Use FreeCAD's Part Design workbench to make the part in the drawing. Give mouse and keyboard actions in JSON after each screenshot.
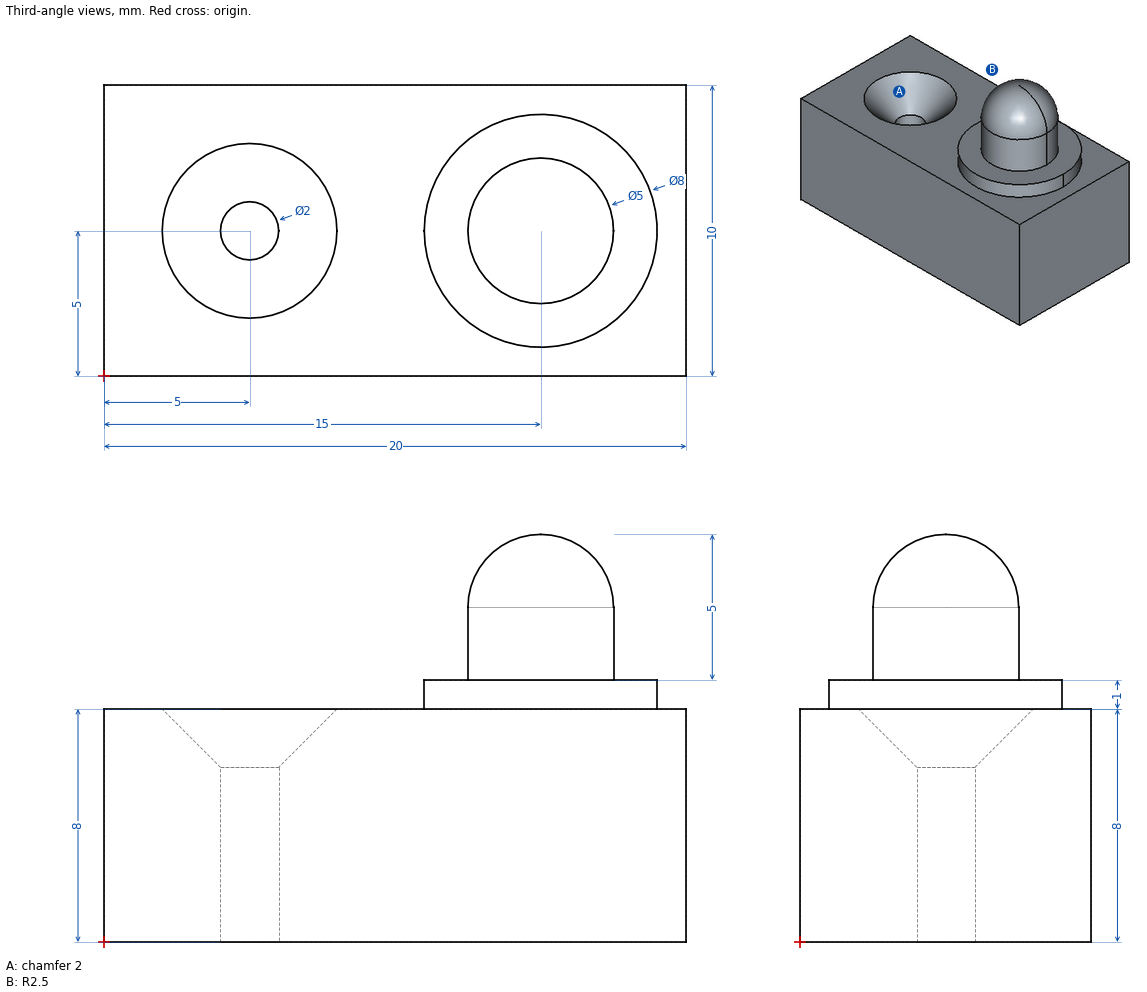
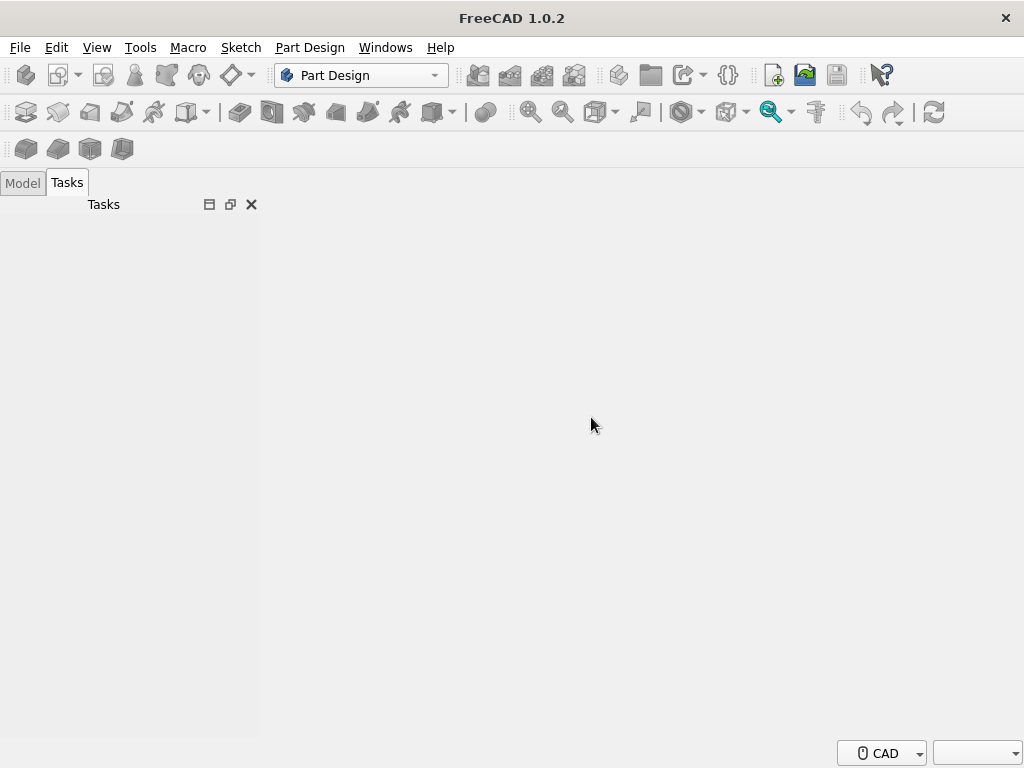
{"action": "left_click", "coordinate": [774, 76]}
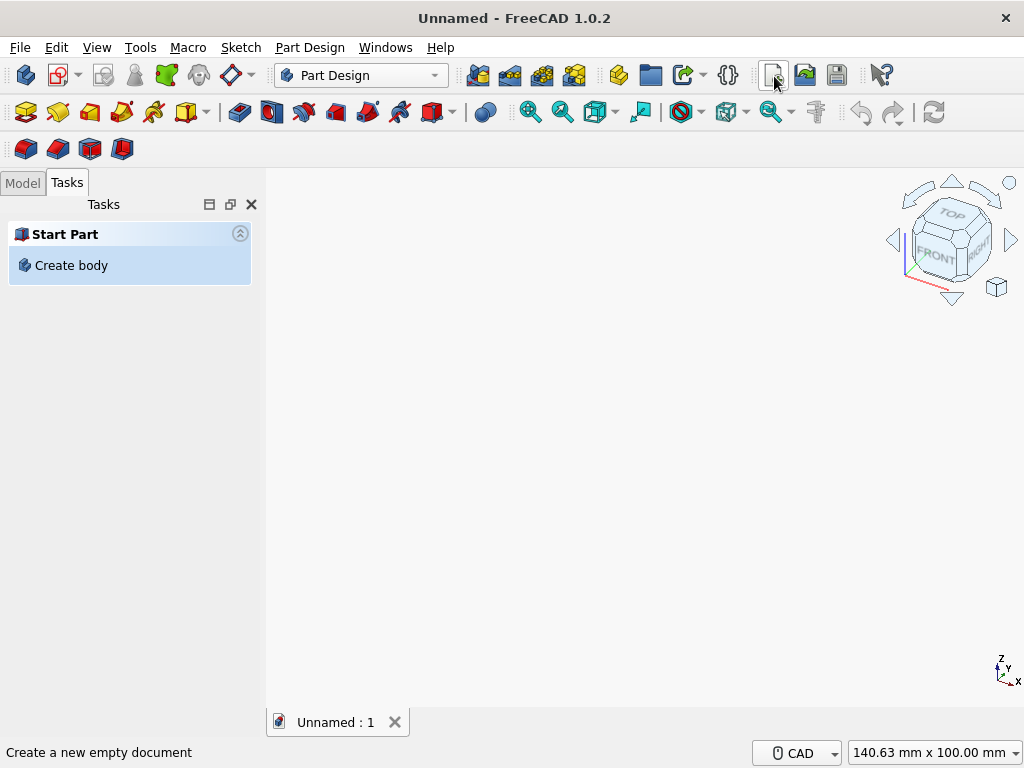
{"action": "left_click", "coordinate": [58, 76]}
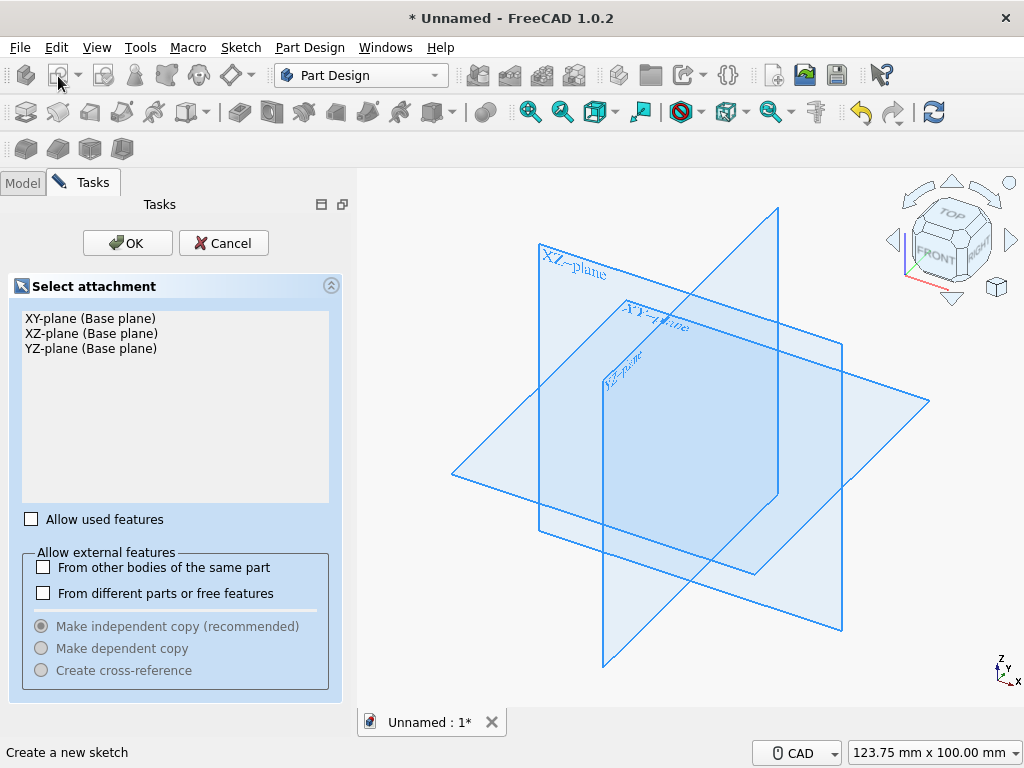
{"action": "left_click", "coordinate": [82, 318]}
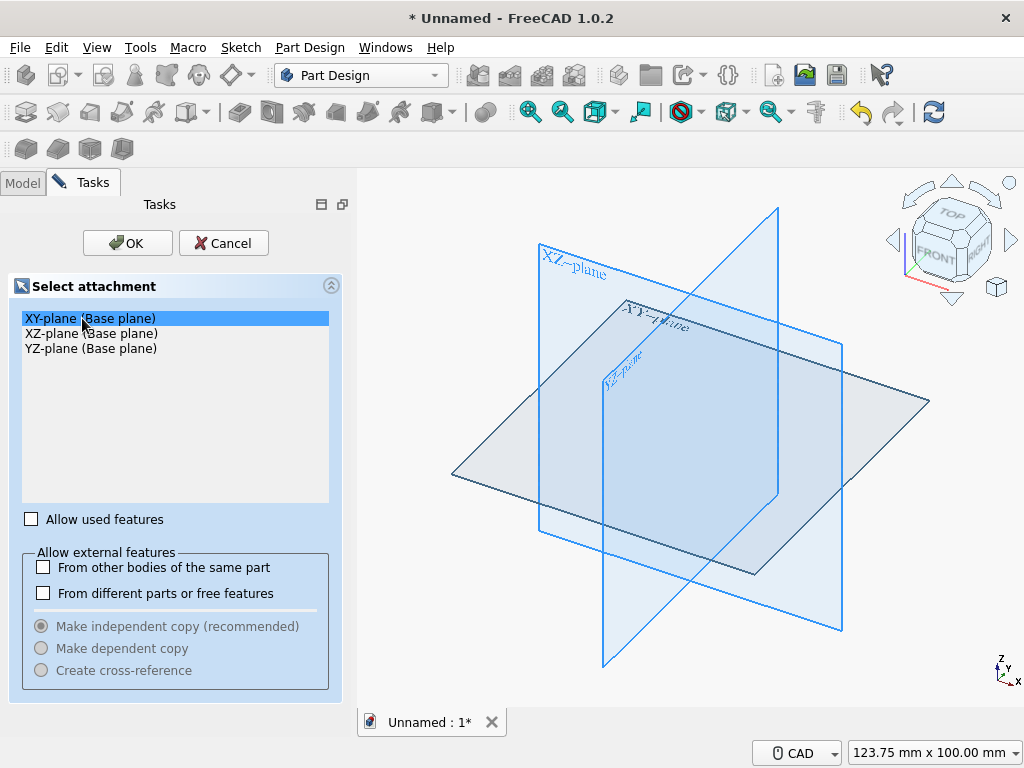
{"action": "left_click", "coordinate": [128, 243]}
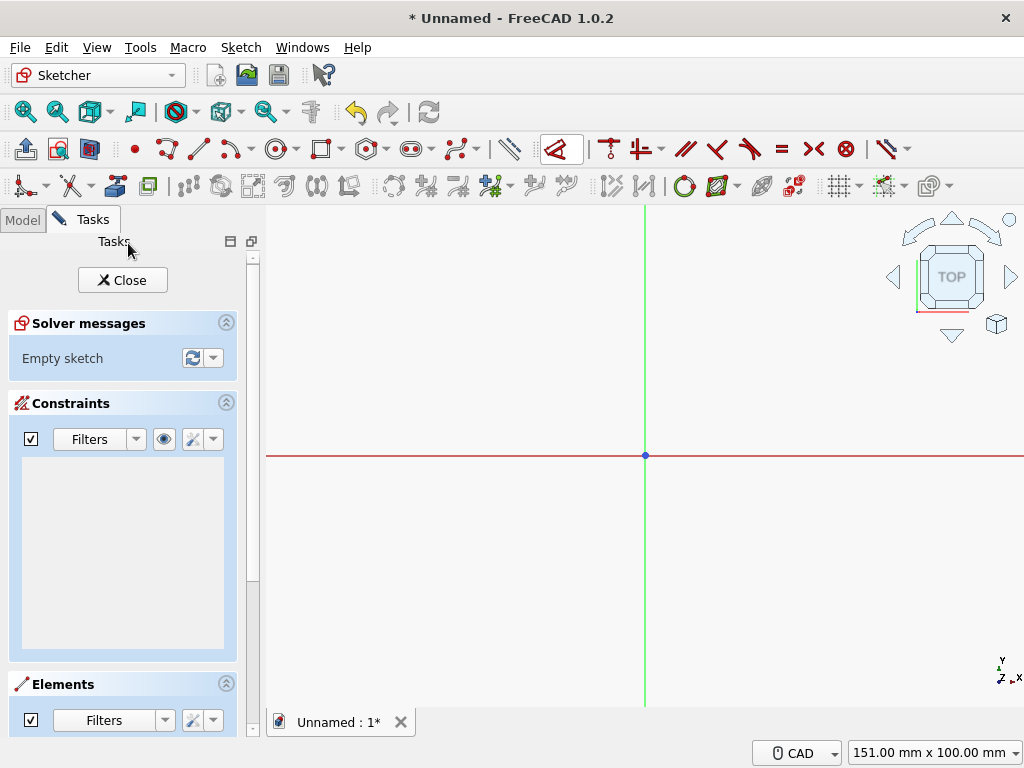
{"action": "scroll", "coordinate": [734, 423], "scroll_direction": "up", "scroll_amount": 7}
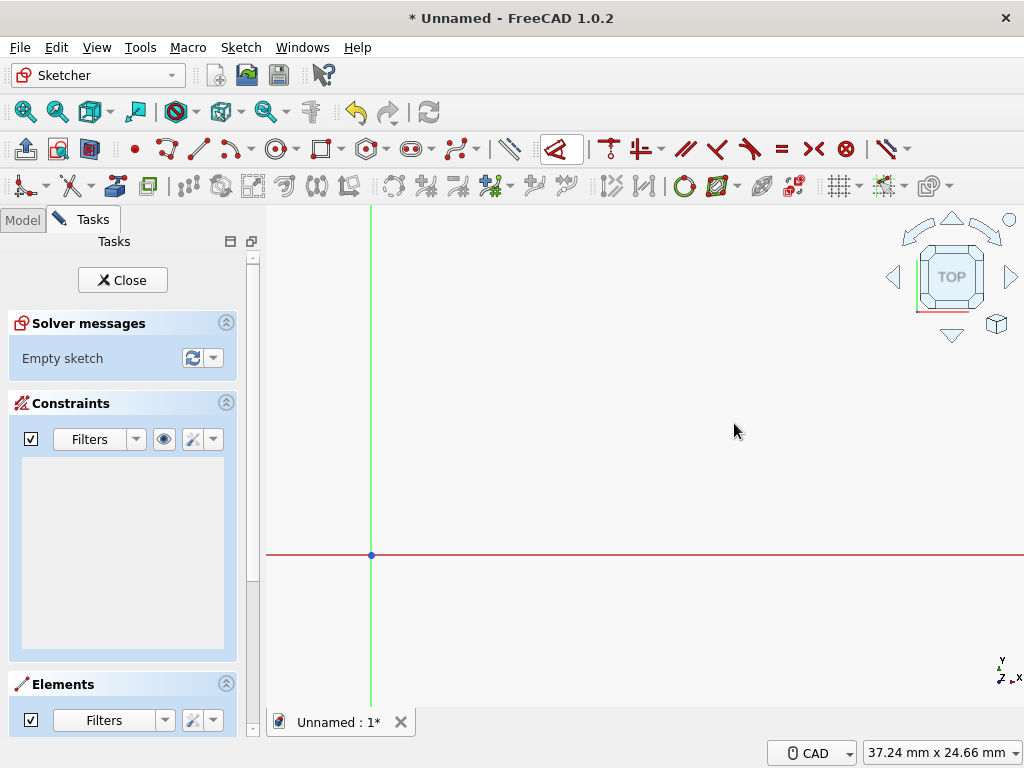
{"action": "left_click", "coordinate": [322, 150]}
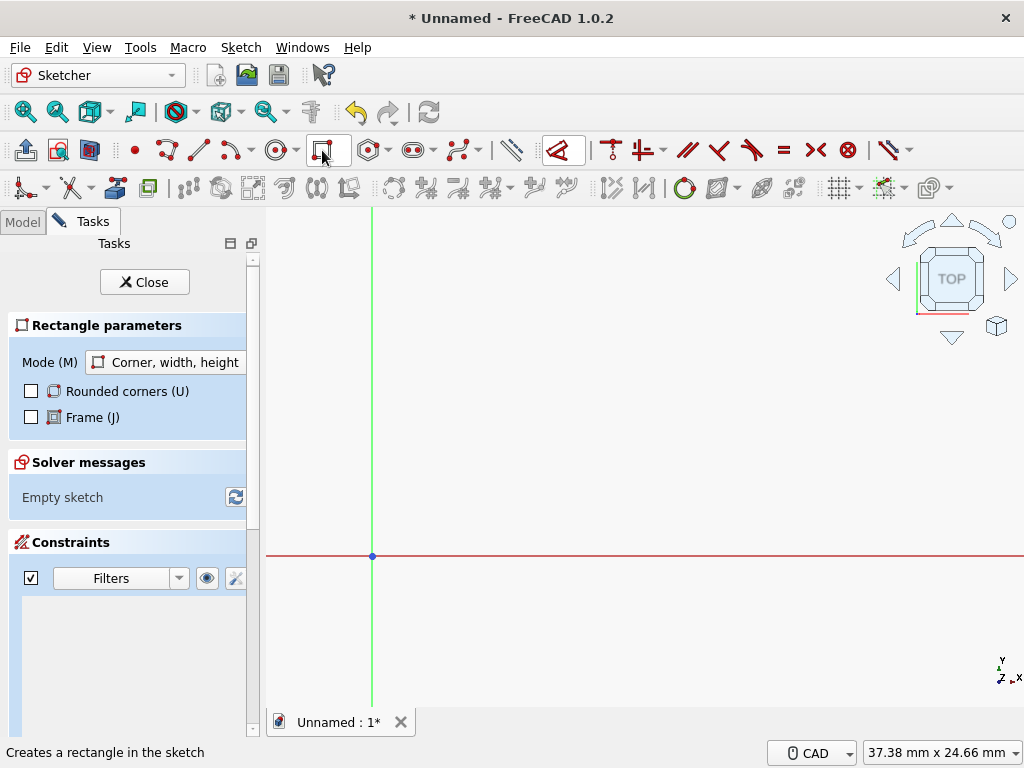
{"action": "left_click", "coordinate": [372, 556]}
{"action": "mouse_move", "coordinate": [778, 353]}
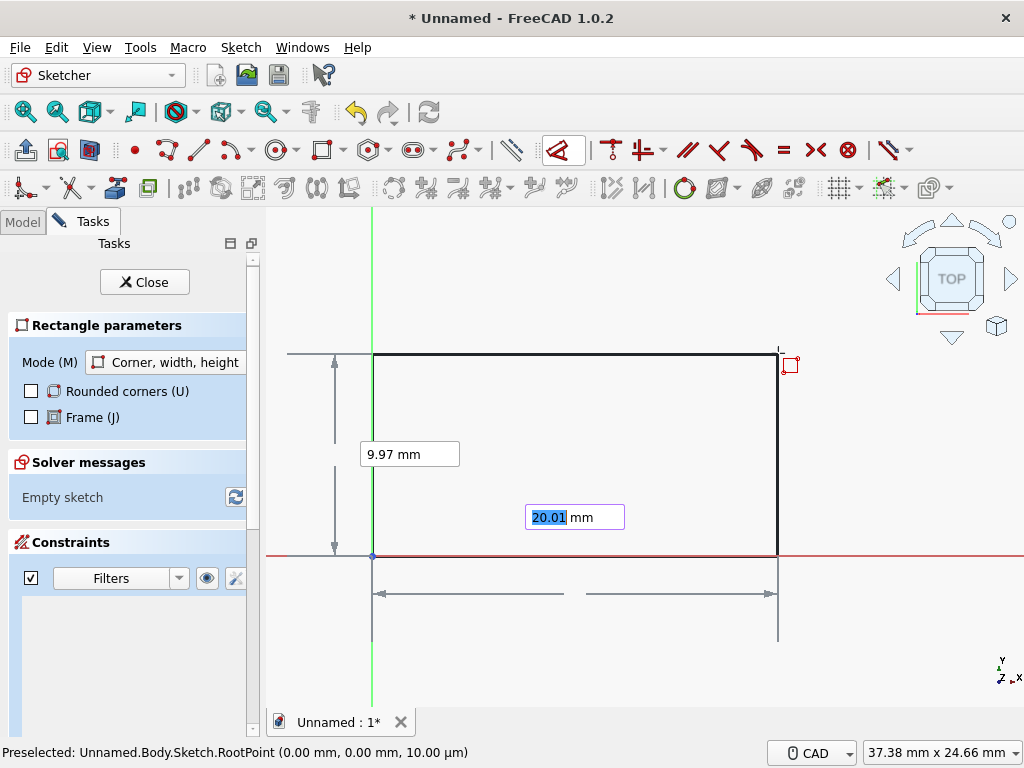
{"action": "type", "text": "20"}
{"action": "key", "text": "Tab"}
{"action": "type", "text": "10"}
{"action": "key", "text": "Return"}
{"action": "key", "text": "Escape"}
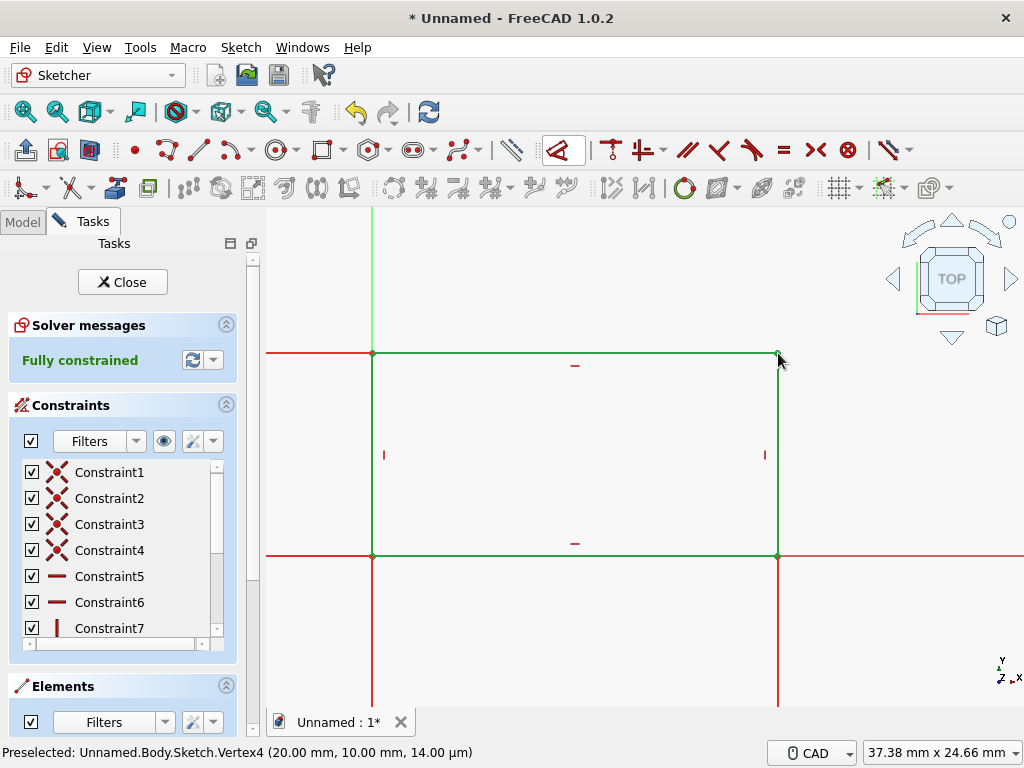
{"action": "left_click", "coordinate": [123, 282]}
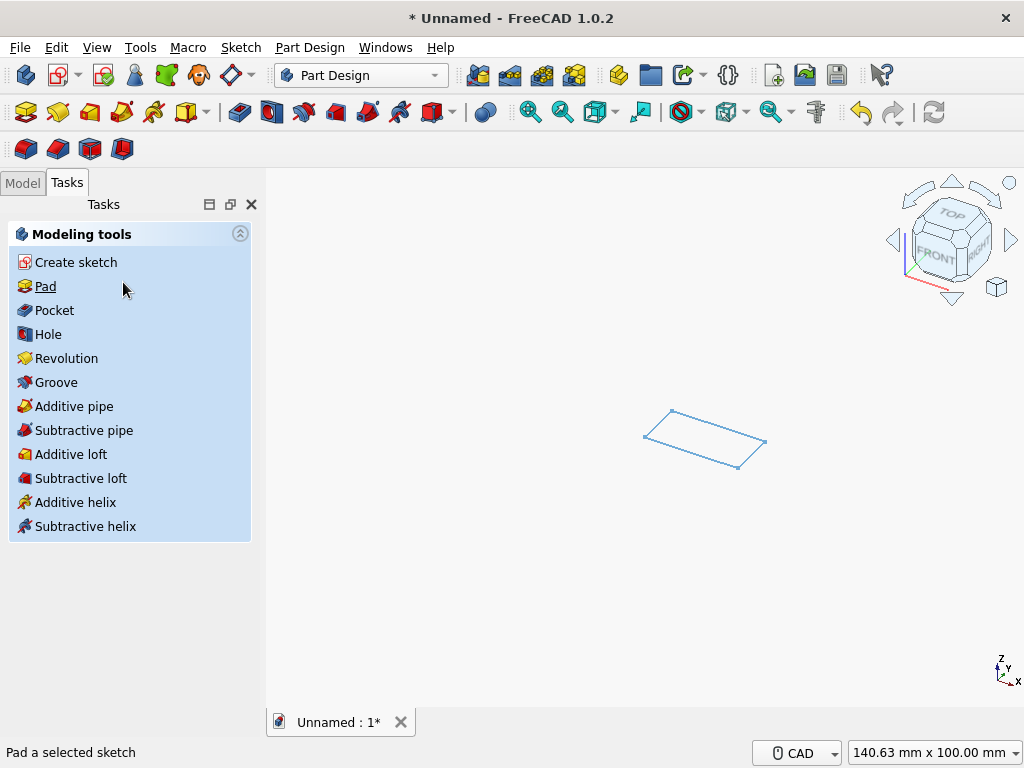
{"action": "left_click", "coordinate": [26, 112]}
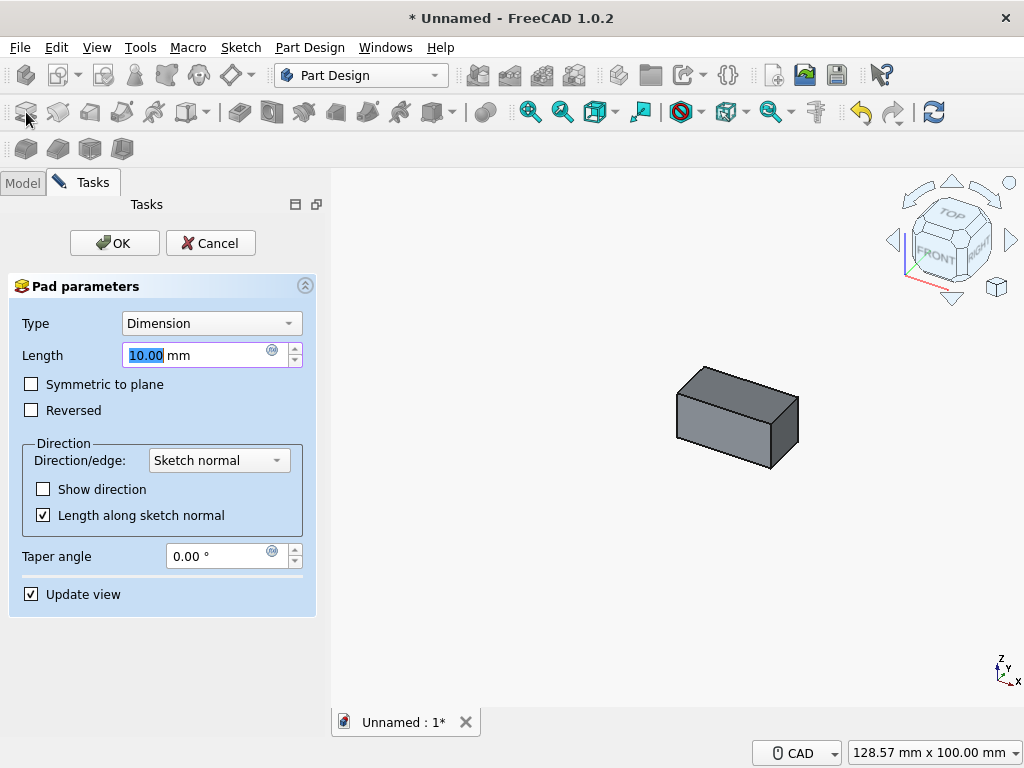
{"action": "type", "text": "8"}
{"action": "key", "text": "Tab"}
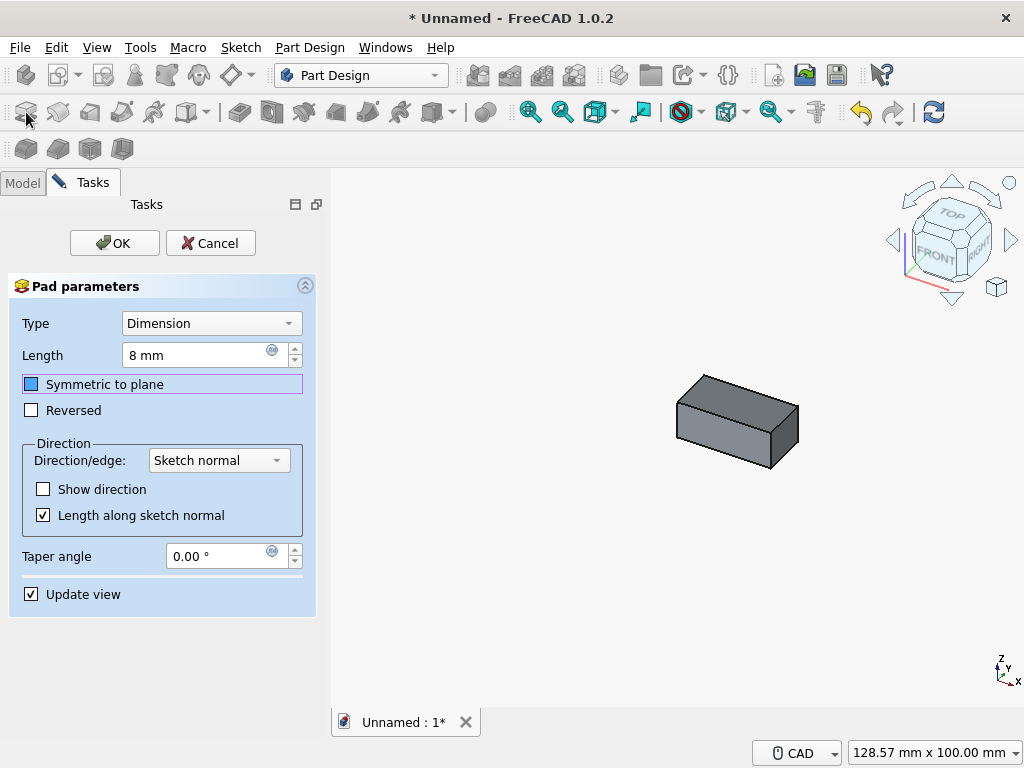
{"action": "left_click", "coordinate": [115, 243]}